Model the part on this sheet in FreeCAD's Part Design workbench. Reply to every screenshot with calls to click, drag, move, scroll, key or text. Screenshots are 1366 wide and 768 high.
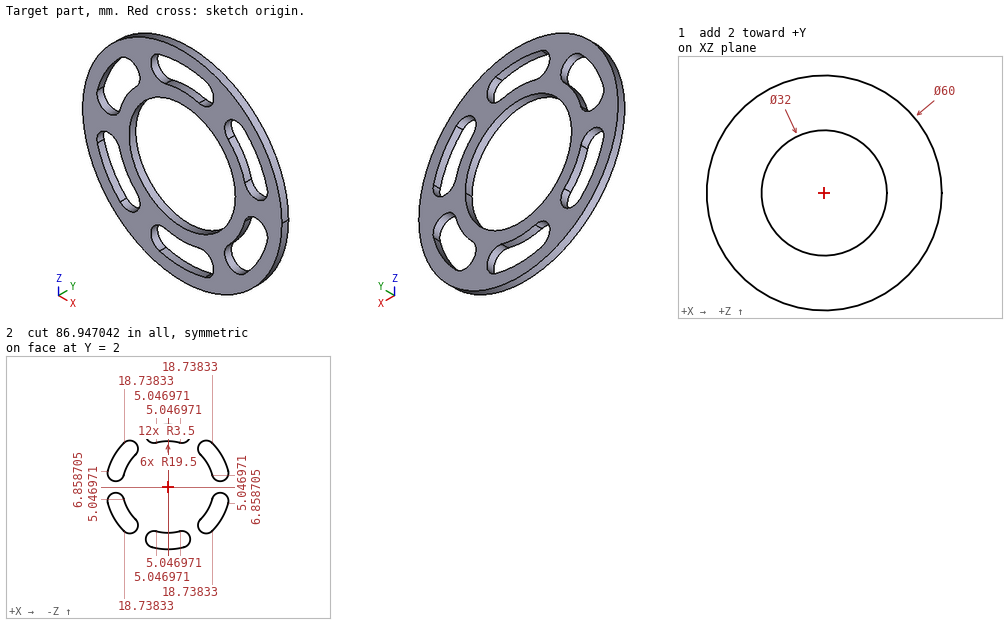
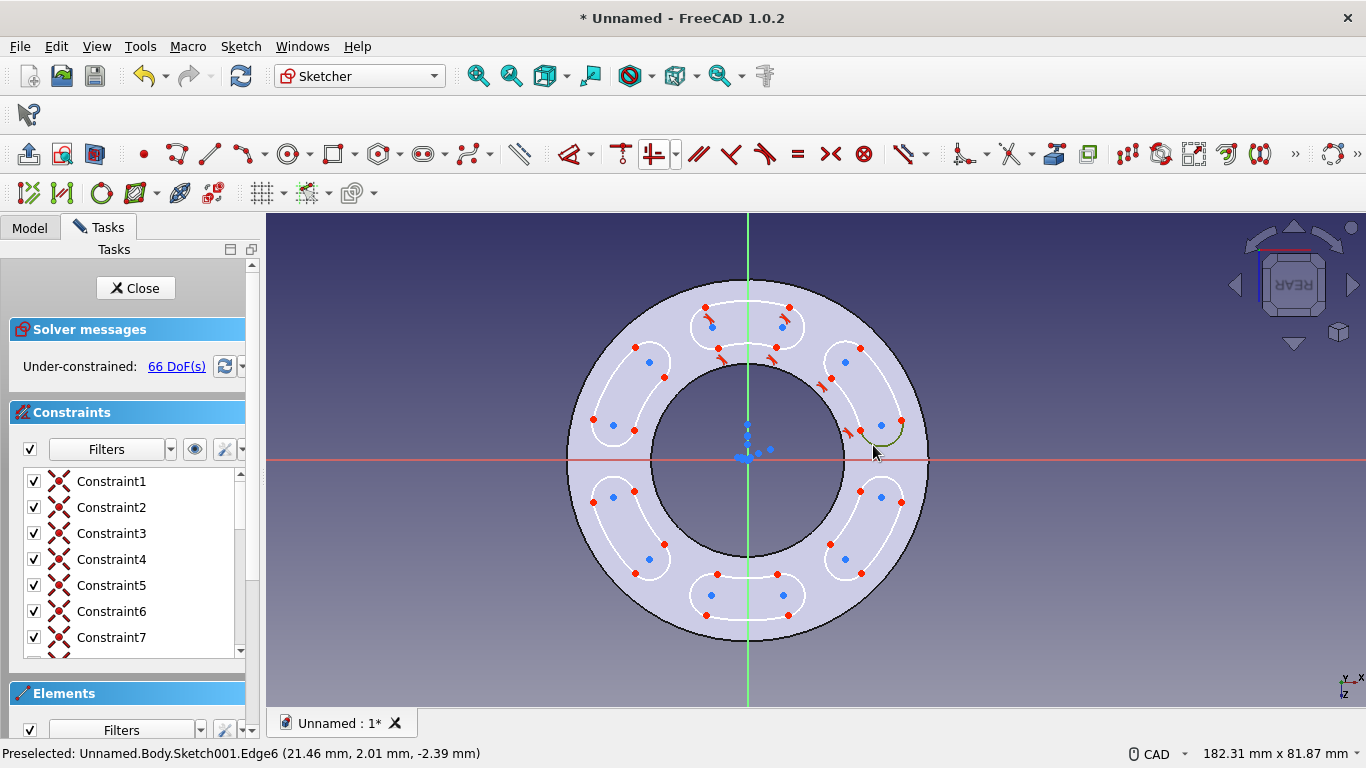
click(894, 396)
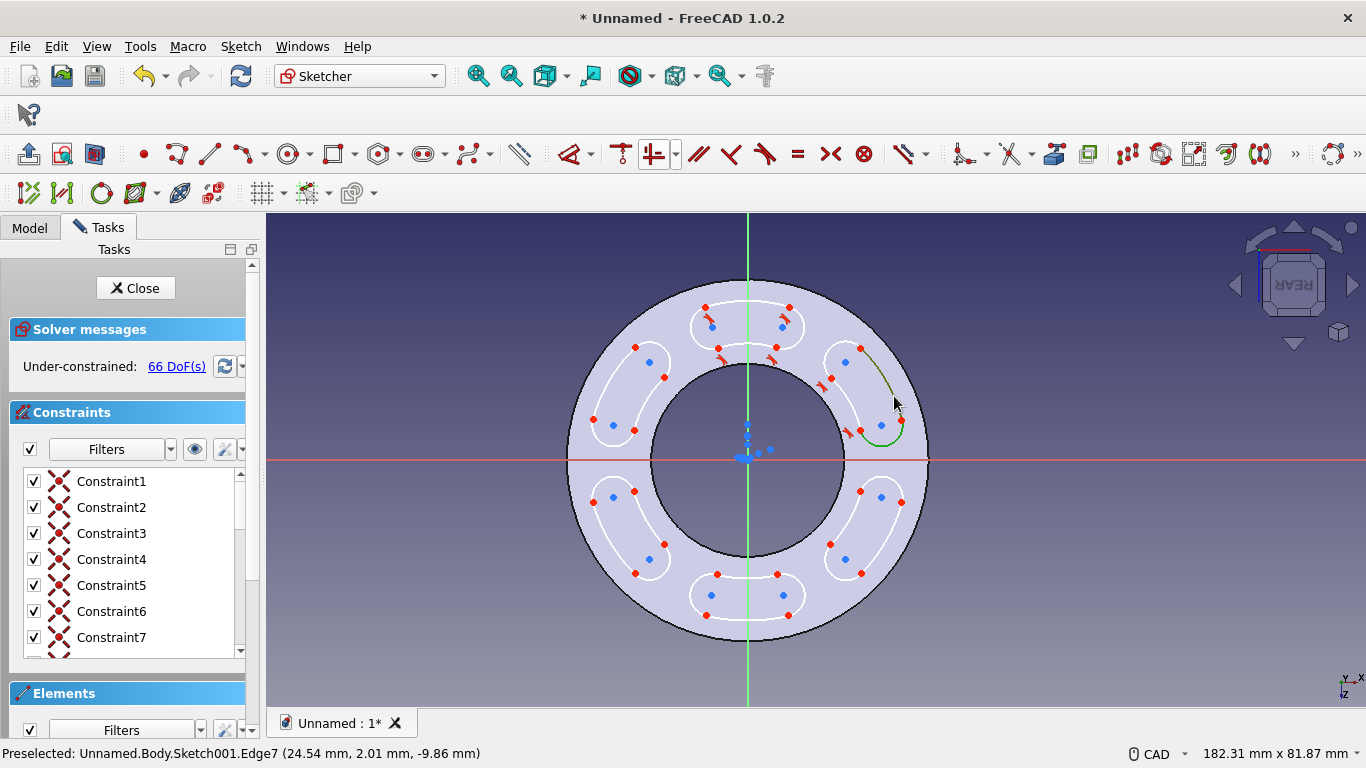
click(765, 154)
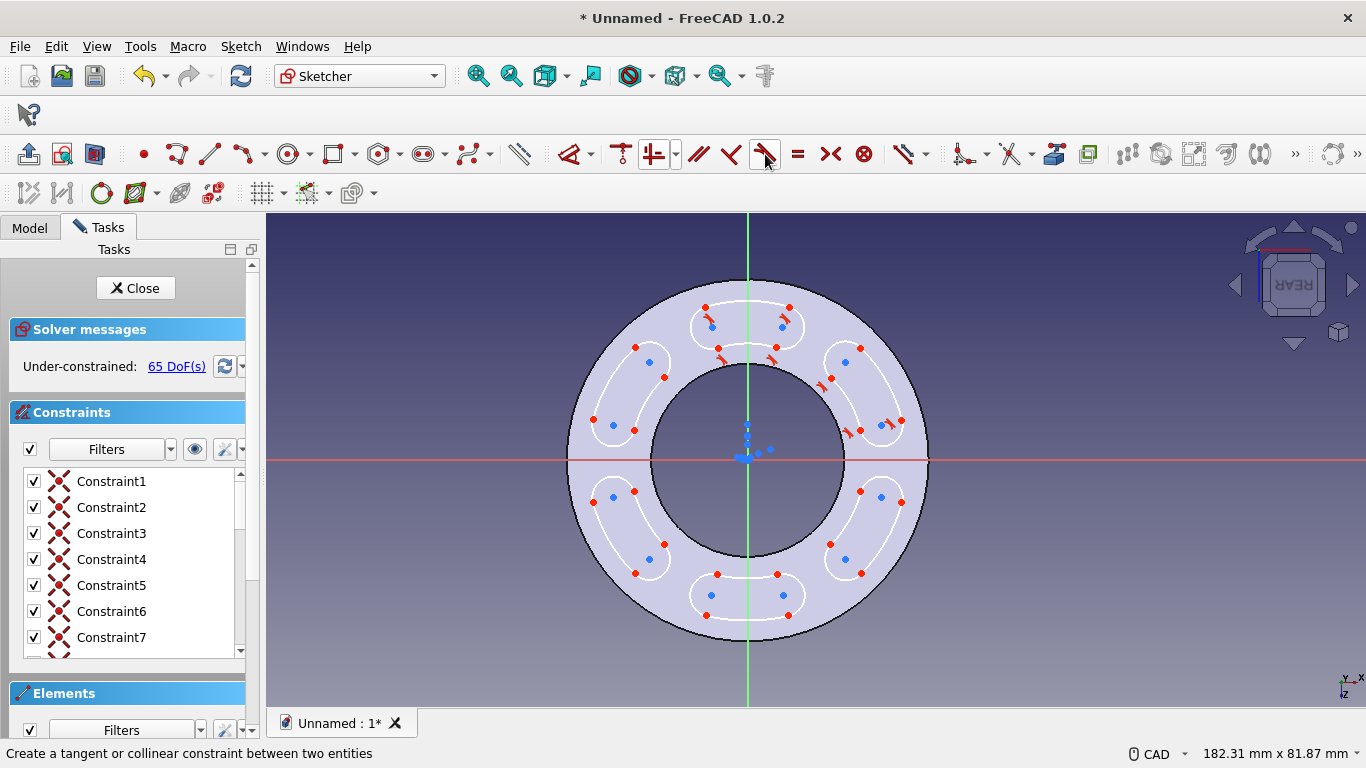
click(894, 396)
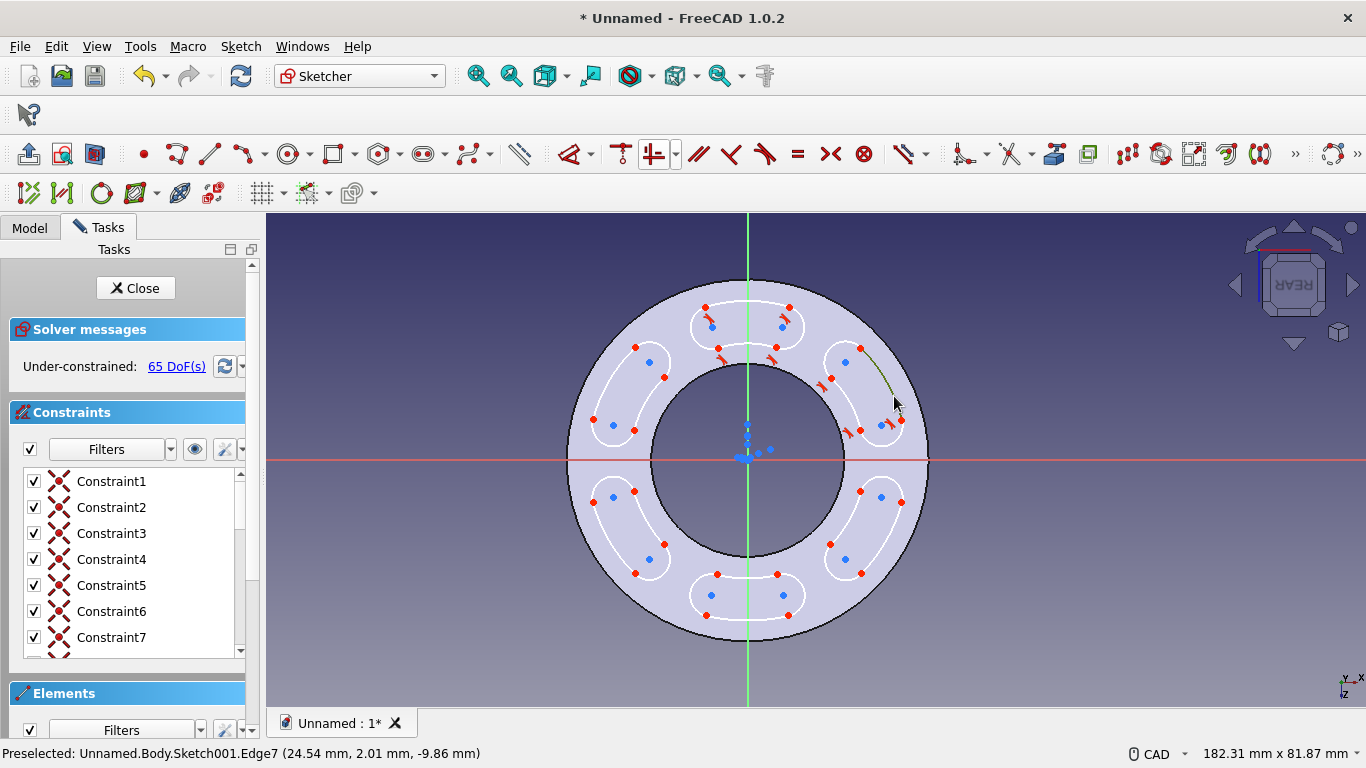
click(843, 342)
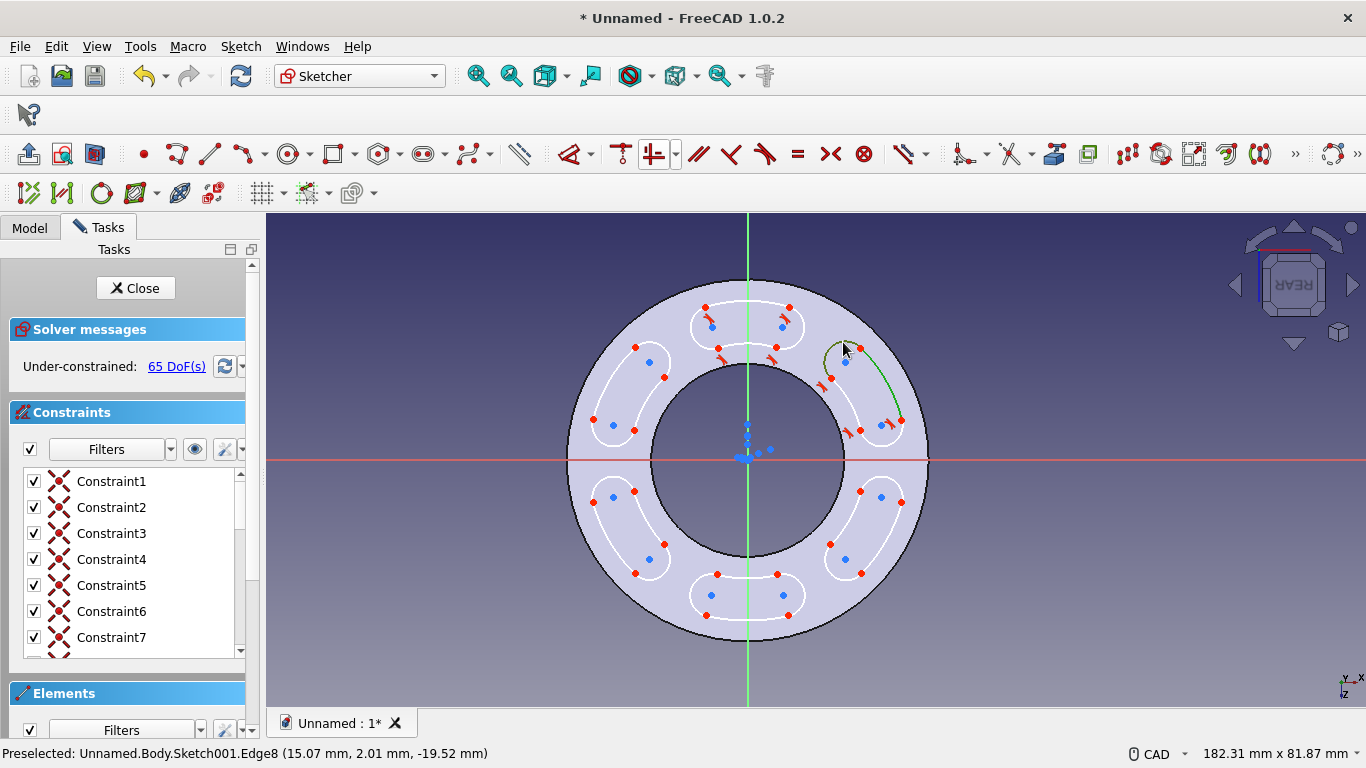
key(t)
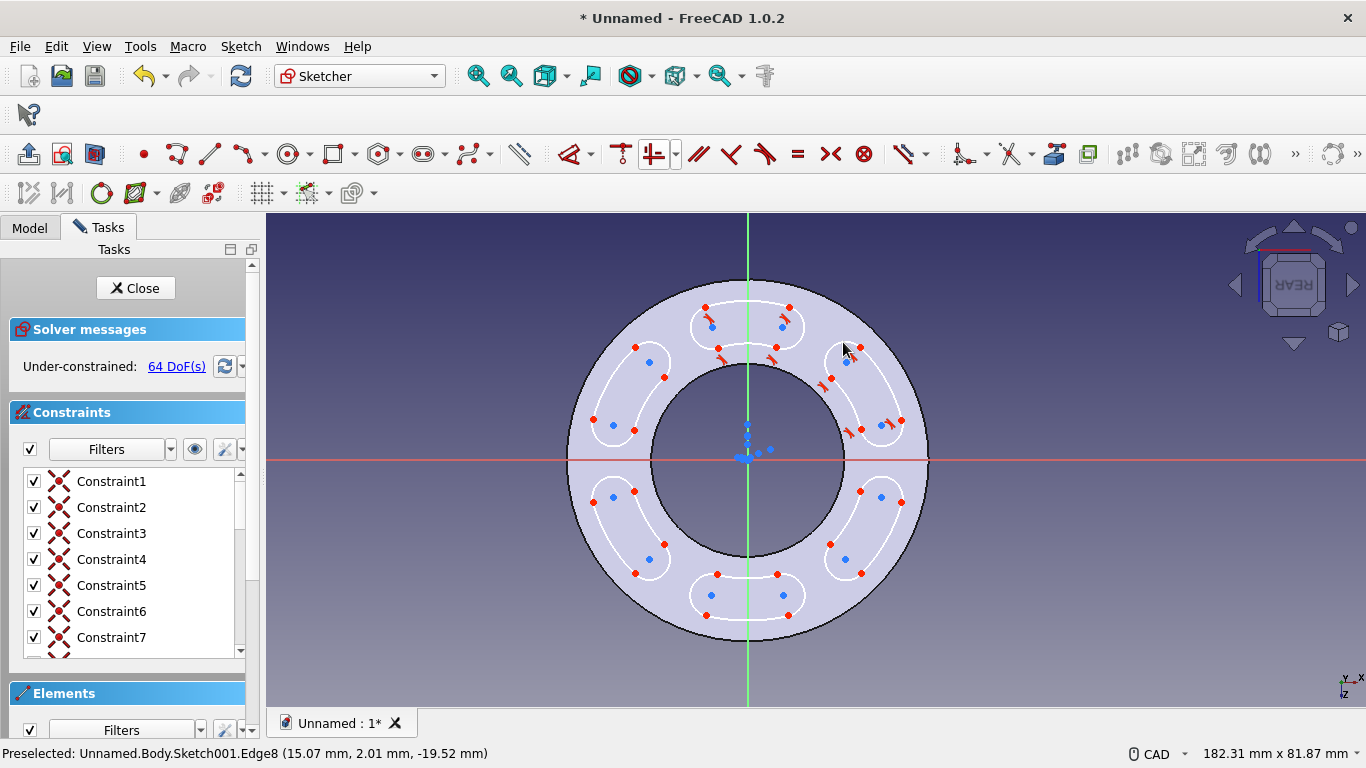
click(825, 563)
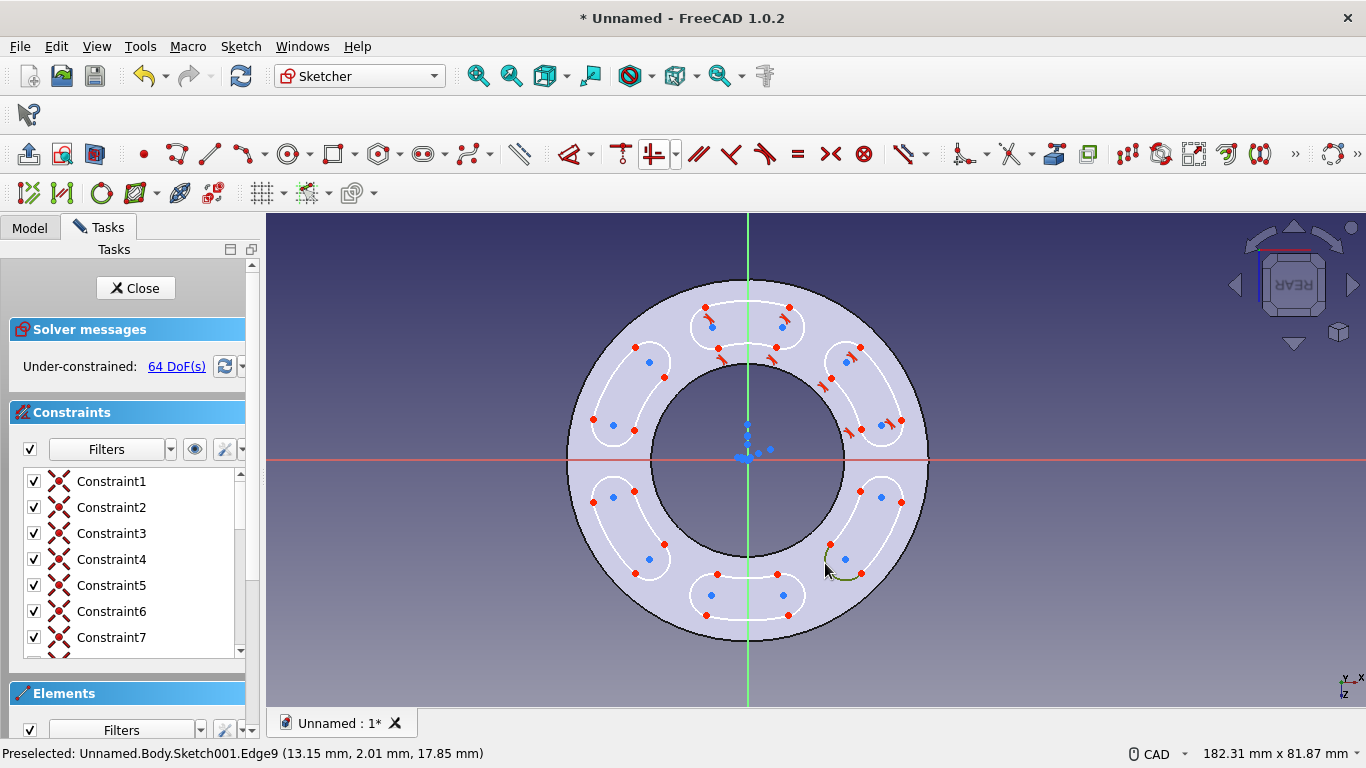
click(877, 555)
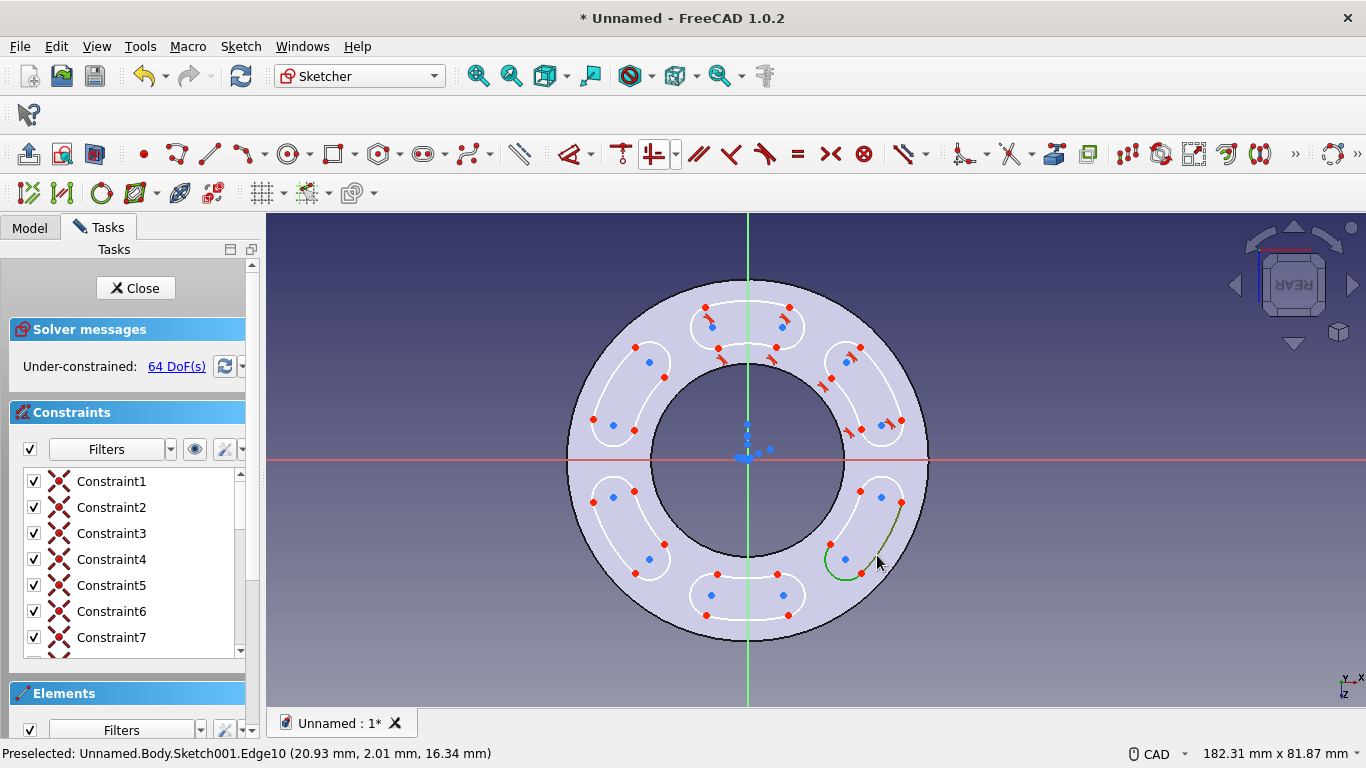
click(765, 154)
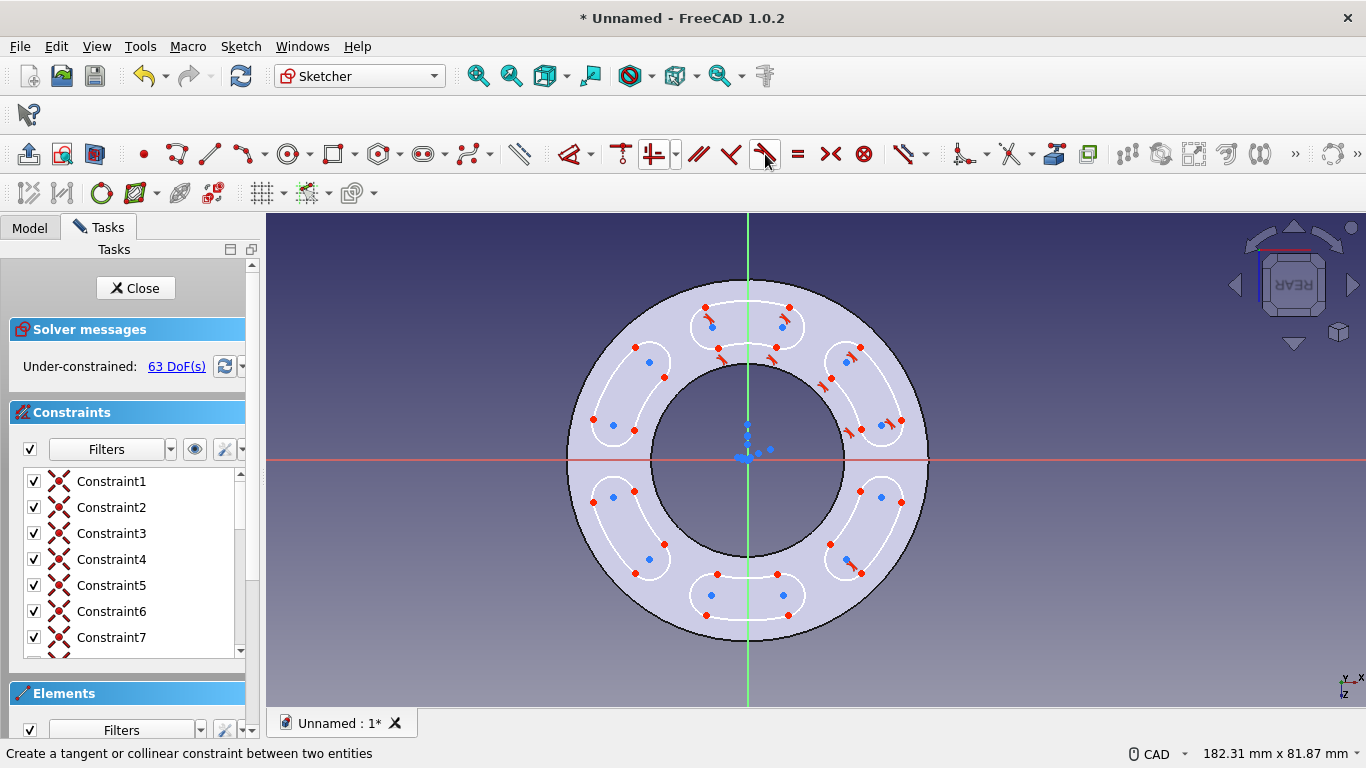
click(826, 563)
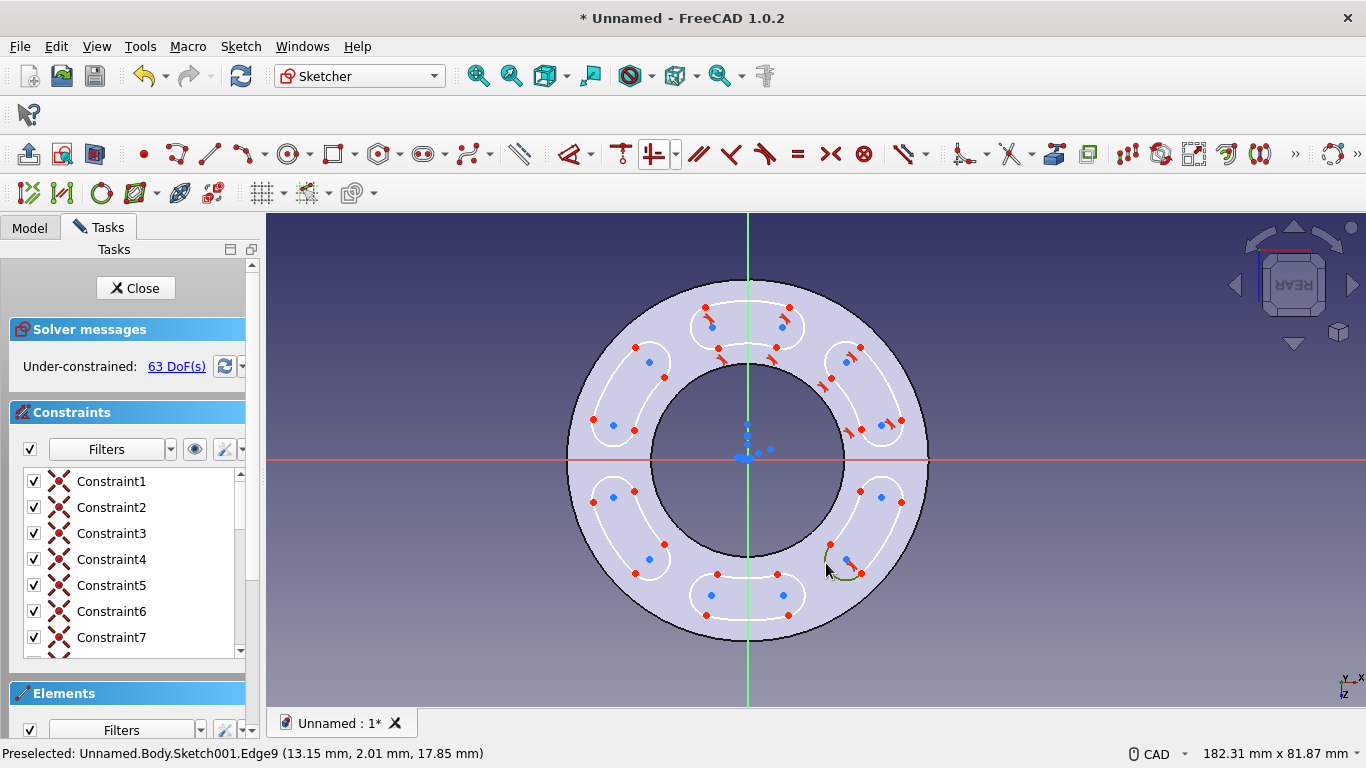
click(843, 531)